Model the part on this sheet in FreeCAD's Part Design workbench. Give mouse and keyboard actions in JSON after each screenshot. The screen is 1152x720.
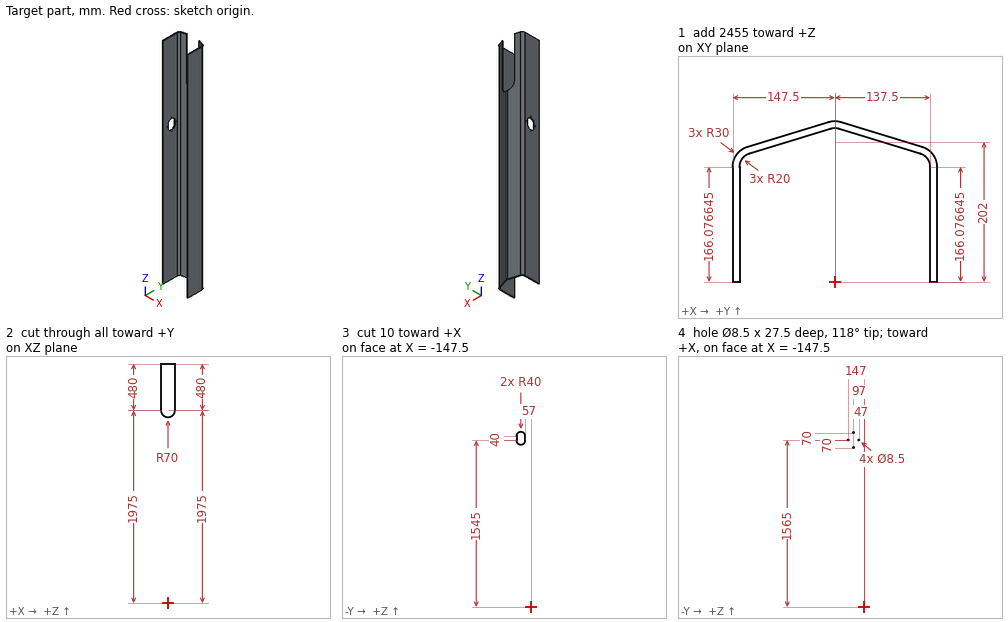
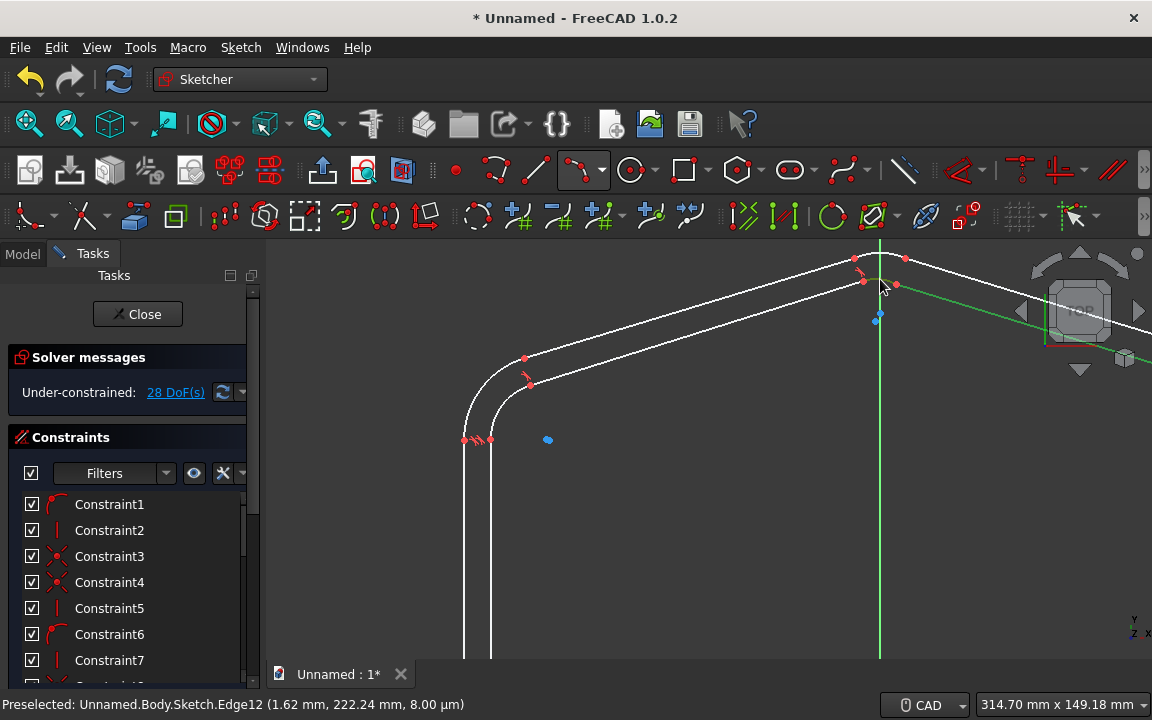
{"action": "key", "text": "t"}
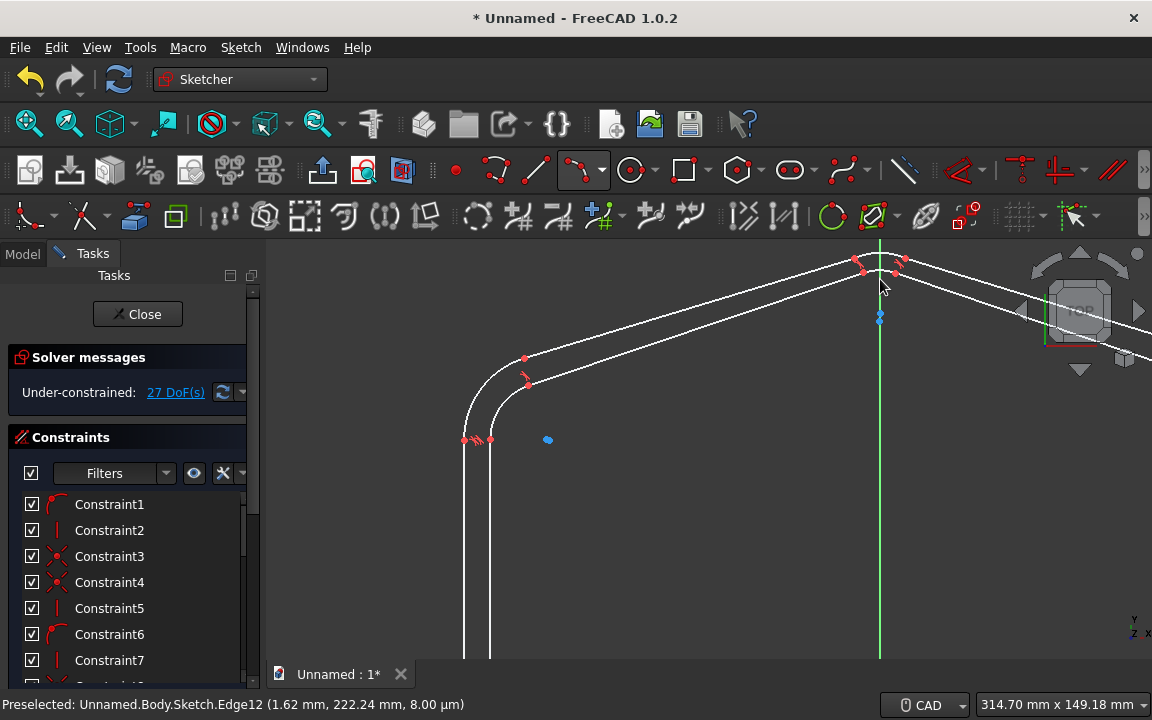
{"action": "left_click", "coordinate": [962, 296]}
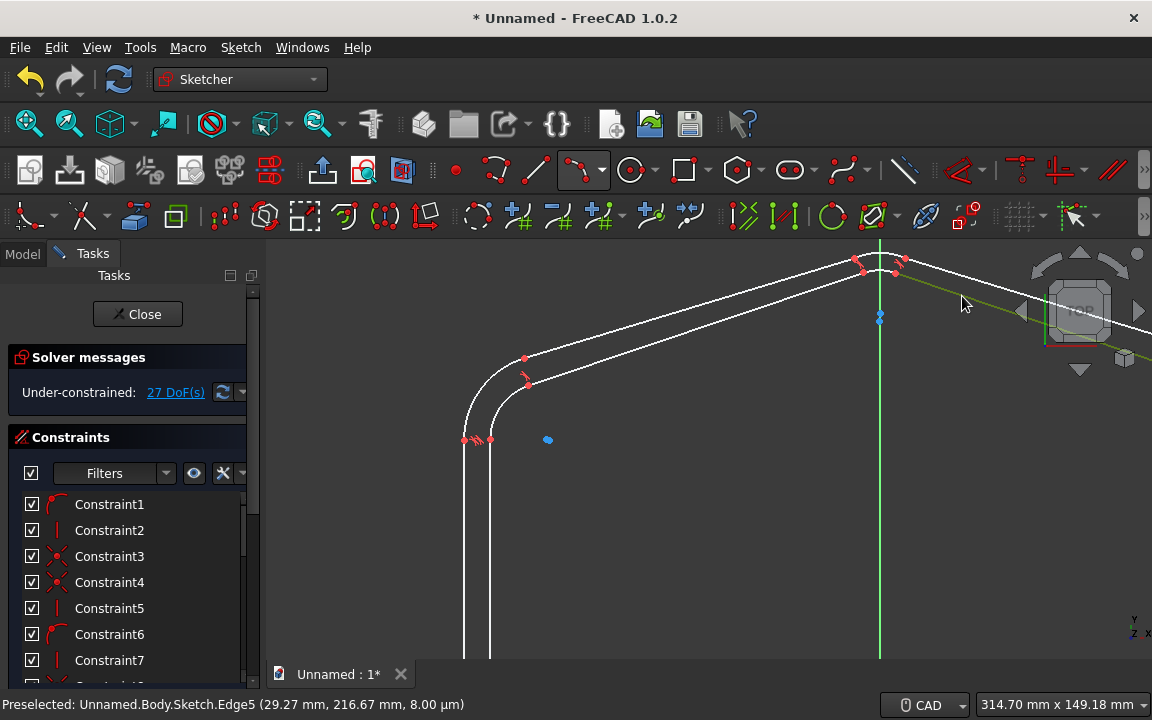
{"action": "scroll", "coordinate": [501, 373], "scroll_direction": "down", "scroll_amount": 5}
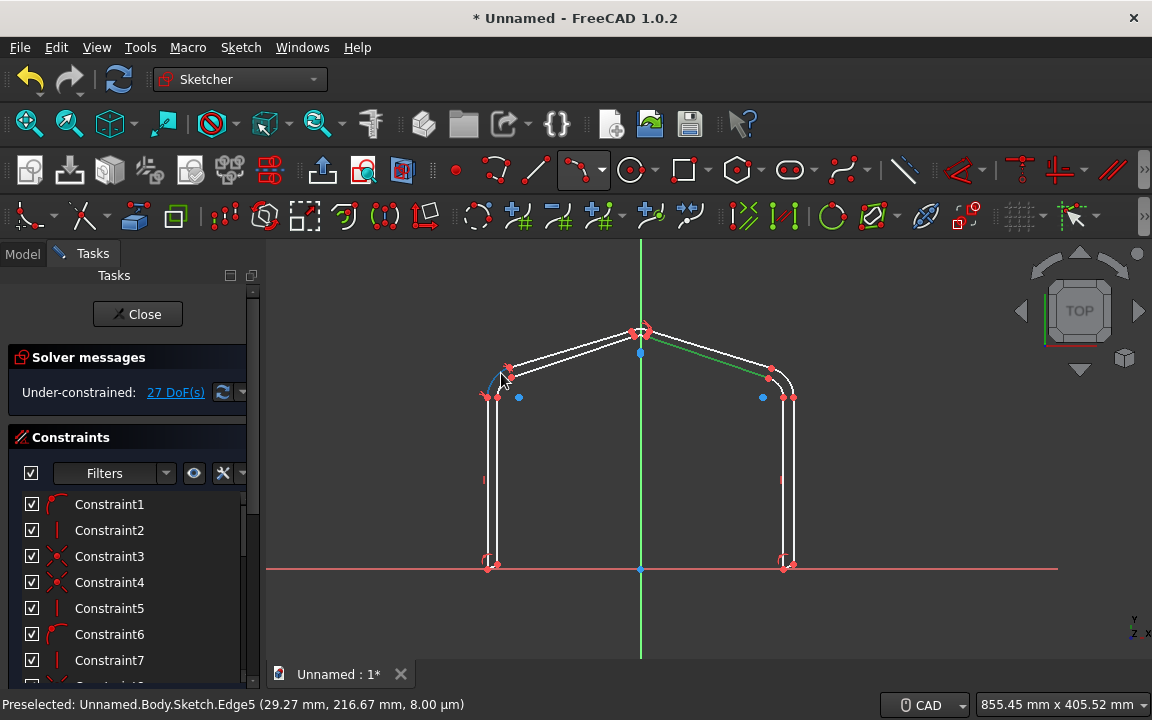
{"action": "scroll", "coordinate": [782, 390], "scroll_direction": "up", "scroll_amount": 3}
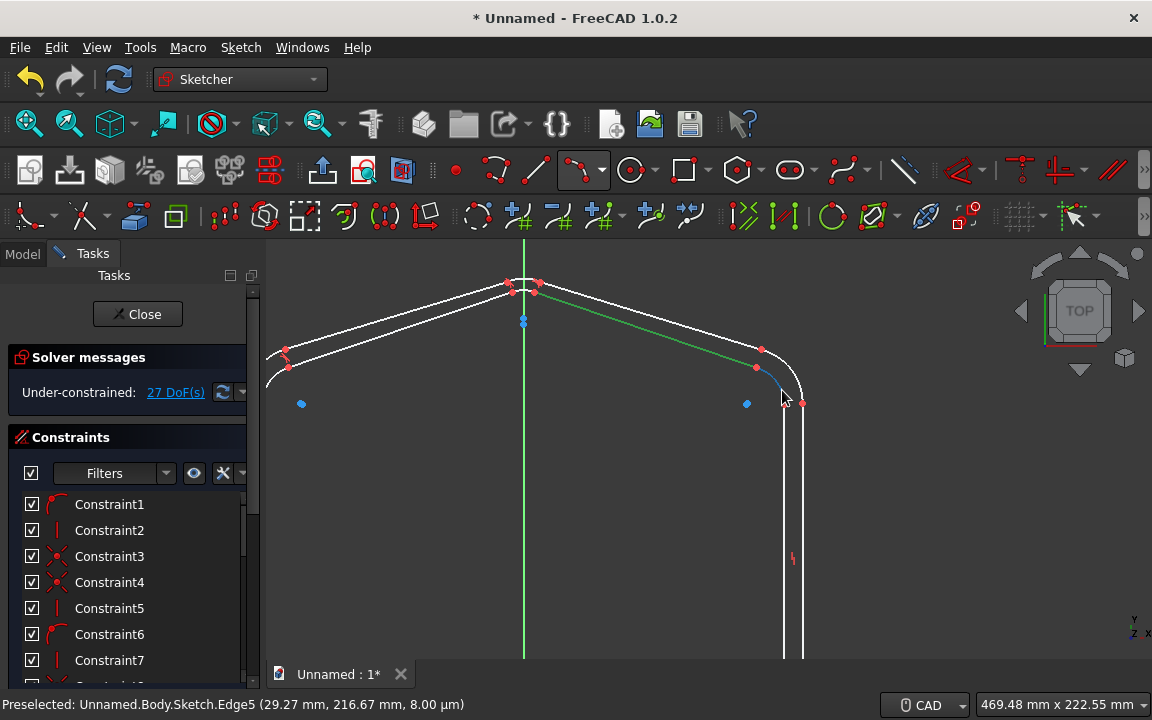
{"action": "left_click", "coordinate": [781, 390]}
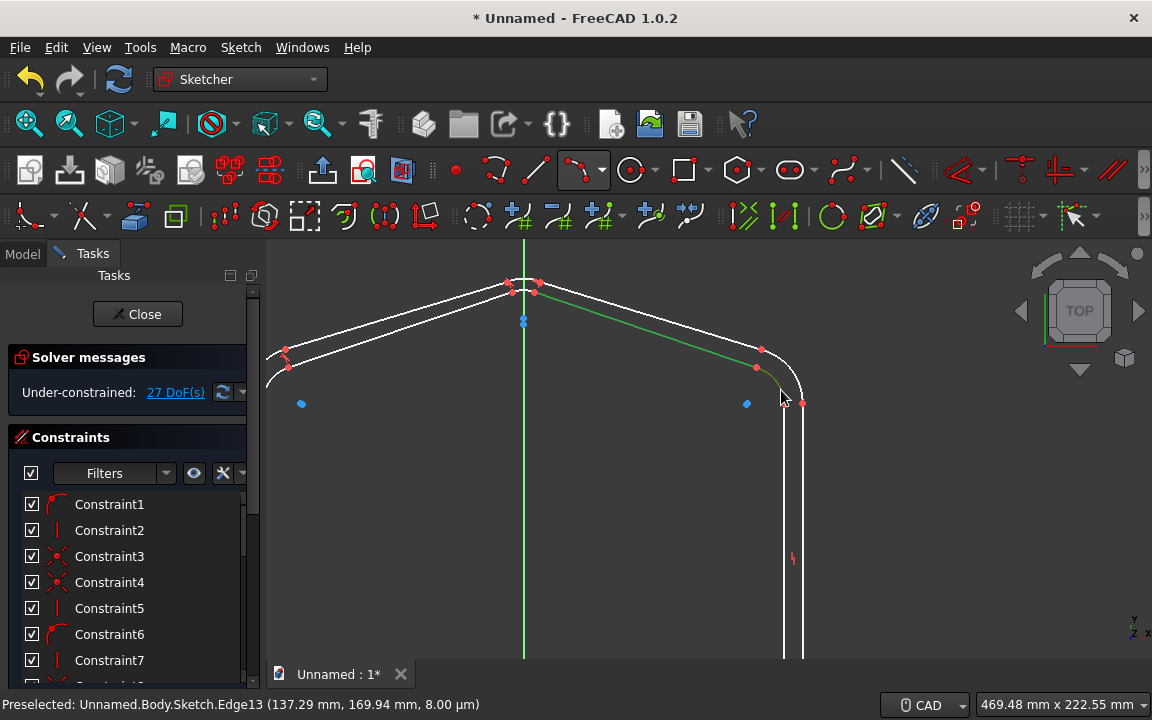
{"action": "key", "text": "t"}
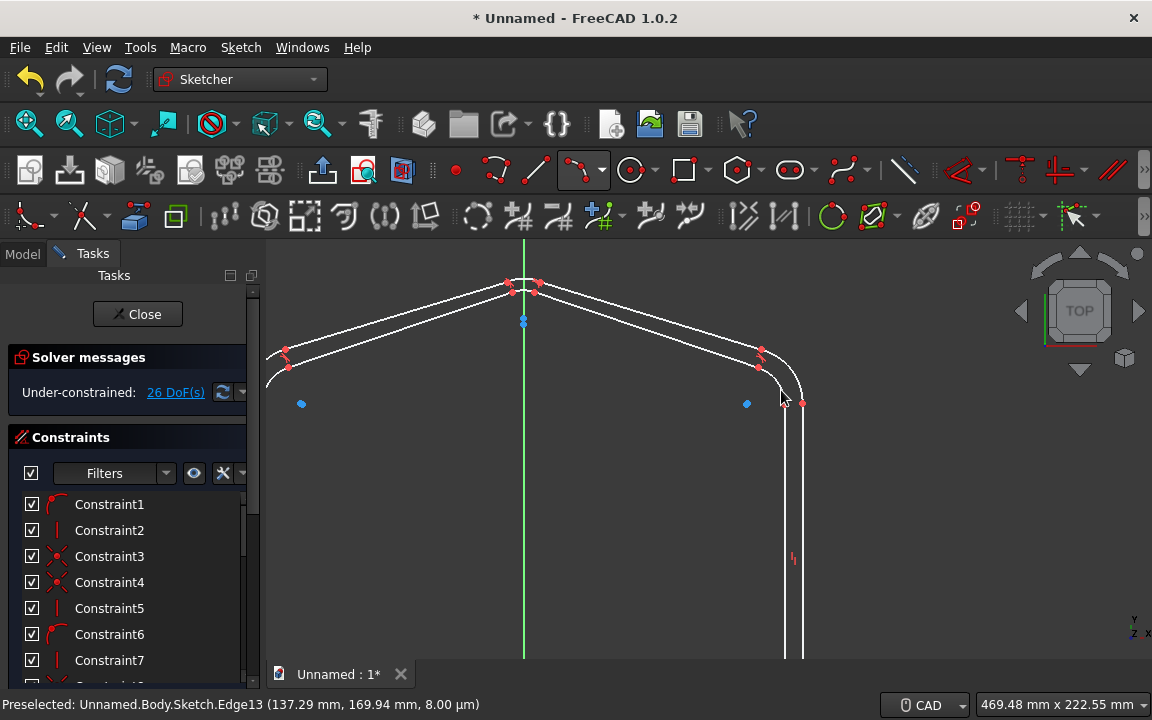
{"action": "left_click", "coordinate": [785, 498]}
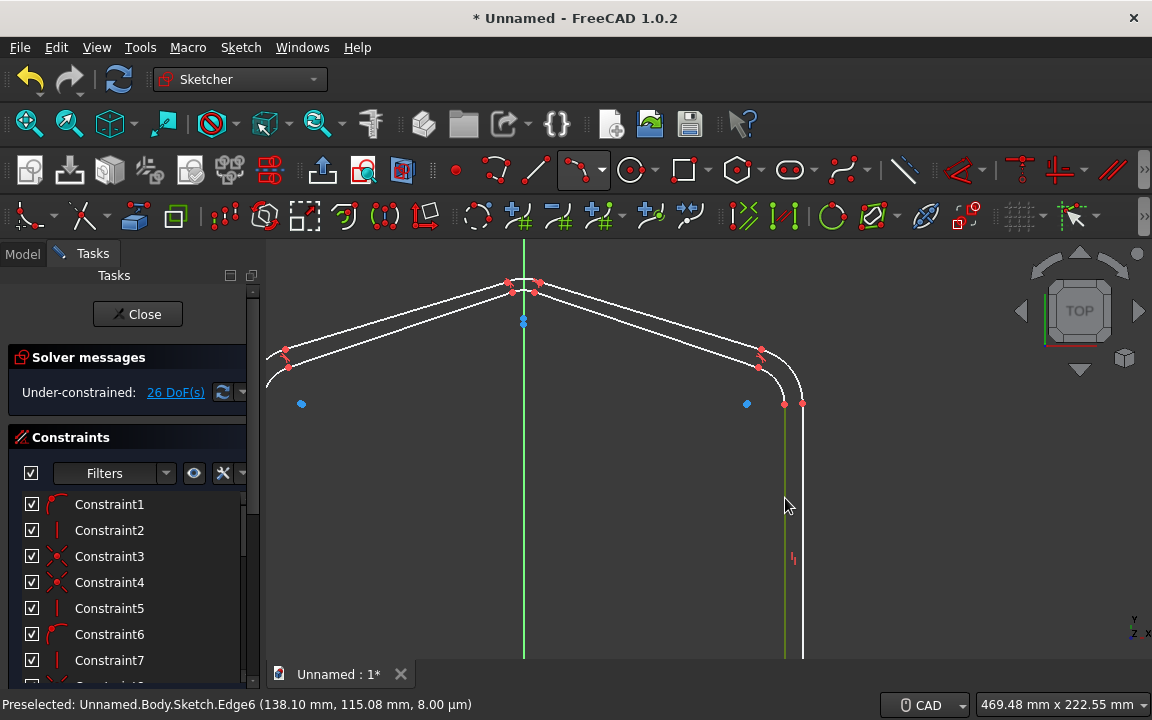
{"action": "left_click", "coordinate": [782, 390]}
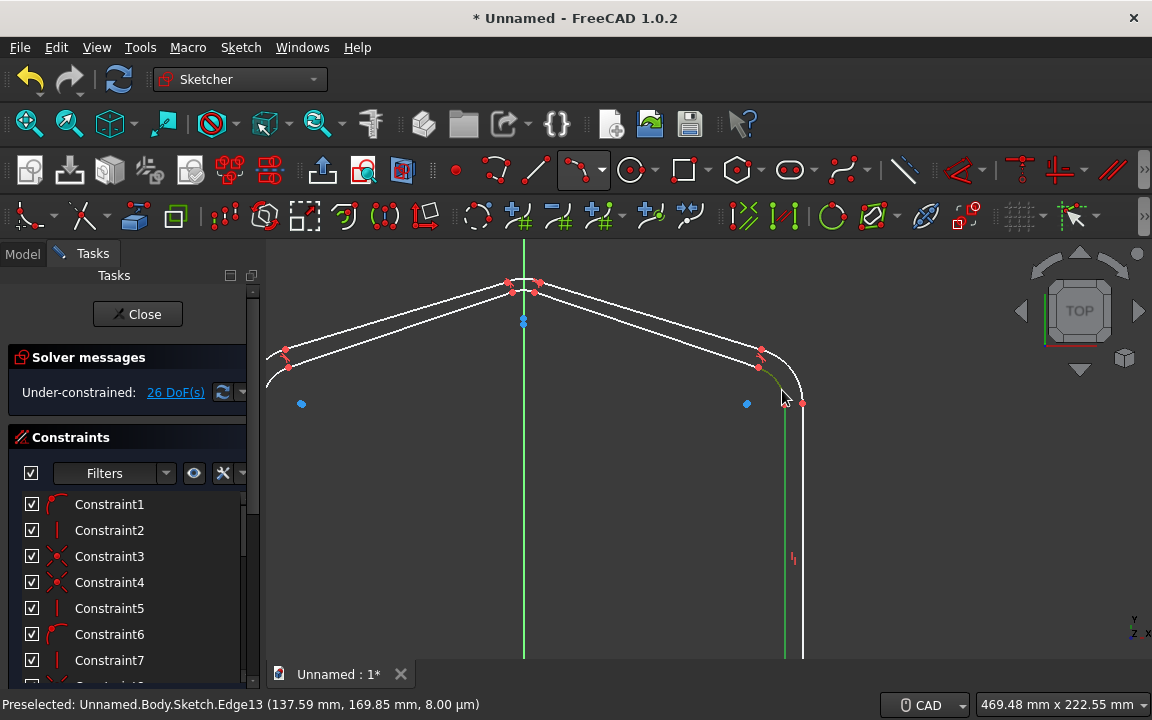
{"action": "key", "text": "t"}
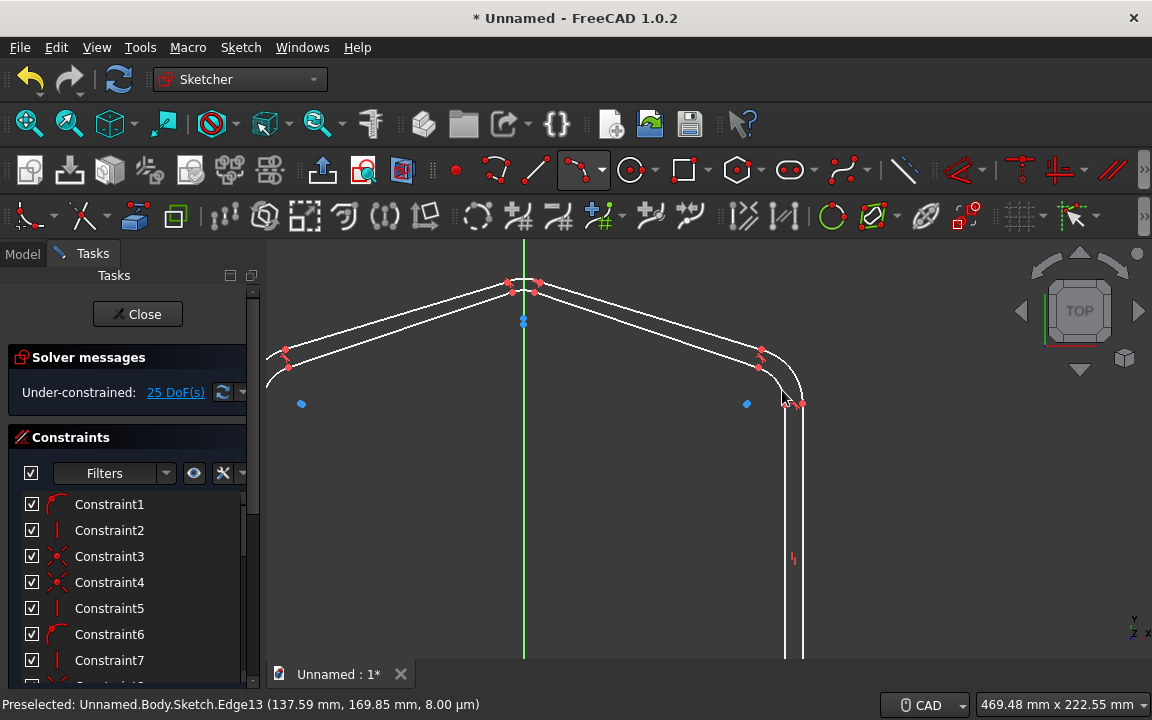
{"action": "left_click", "coordinate": [803, 617]}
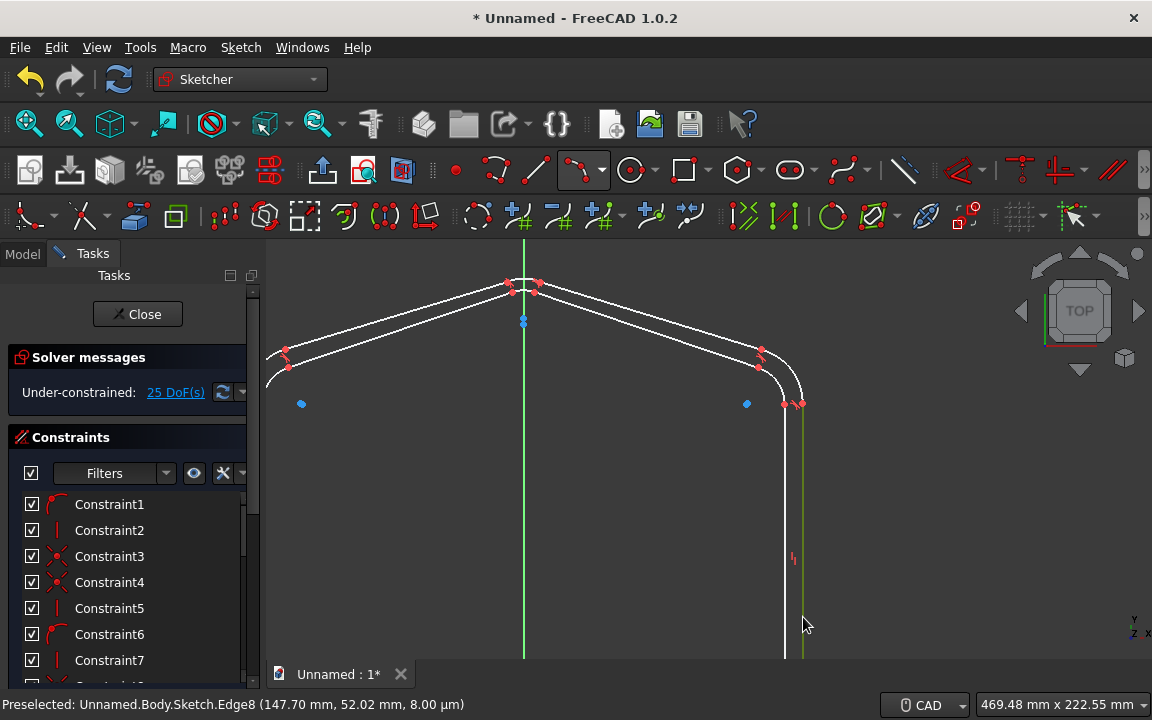
{"action": "left_click", "coordinate": [799, 382]}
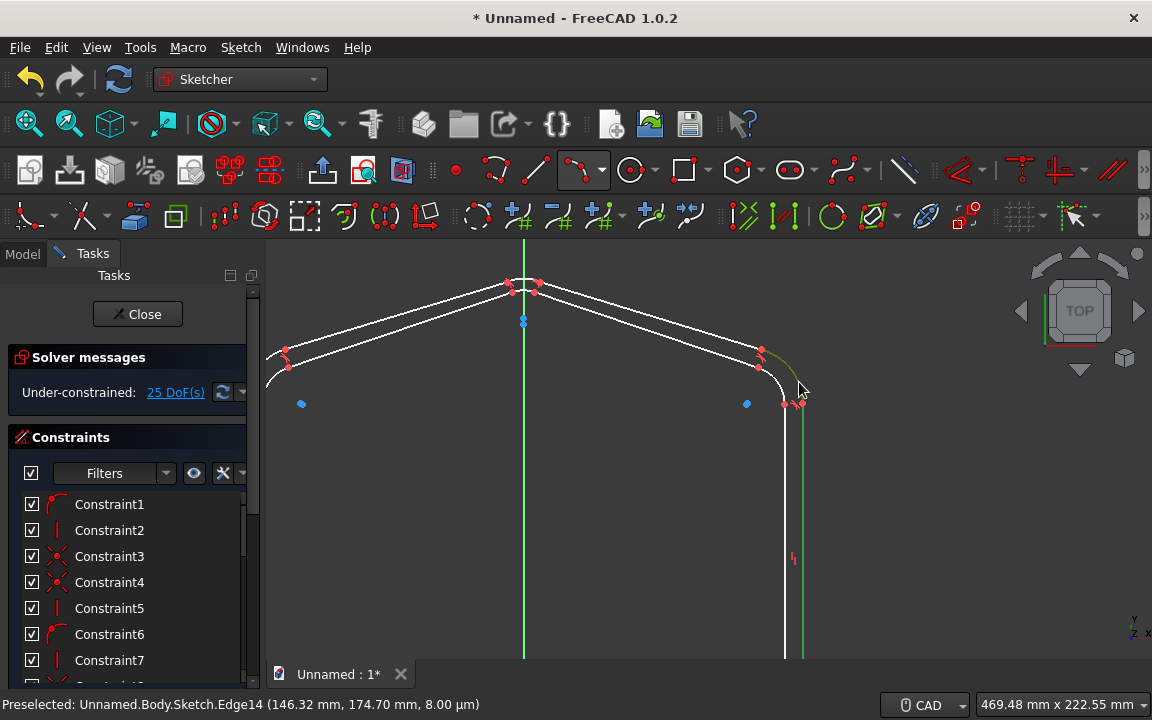
{"action": "key", "text": "t"}